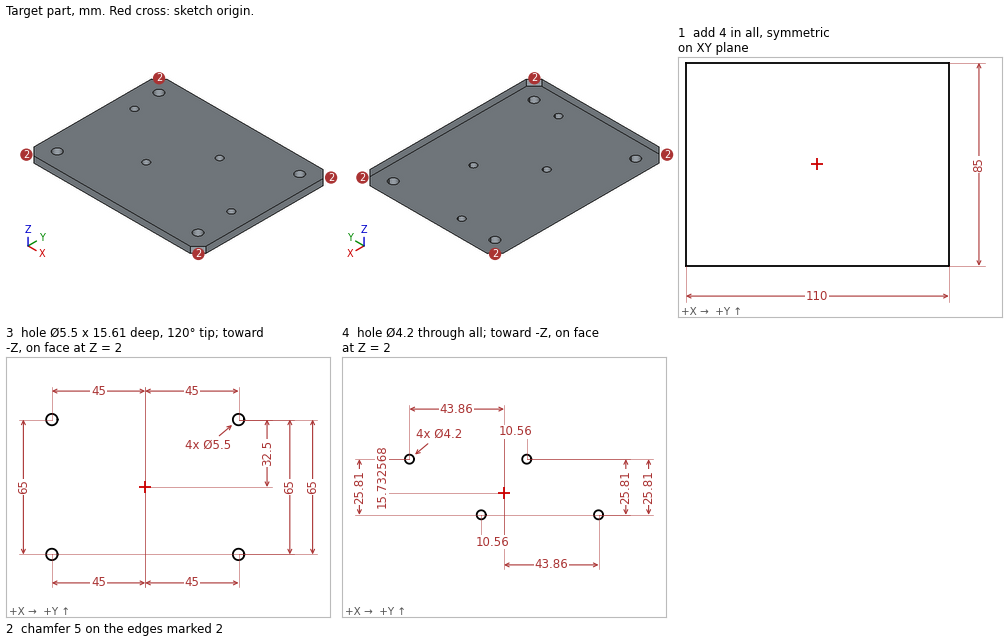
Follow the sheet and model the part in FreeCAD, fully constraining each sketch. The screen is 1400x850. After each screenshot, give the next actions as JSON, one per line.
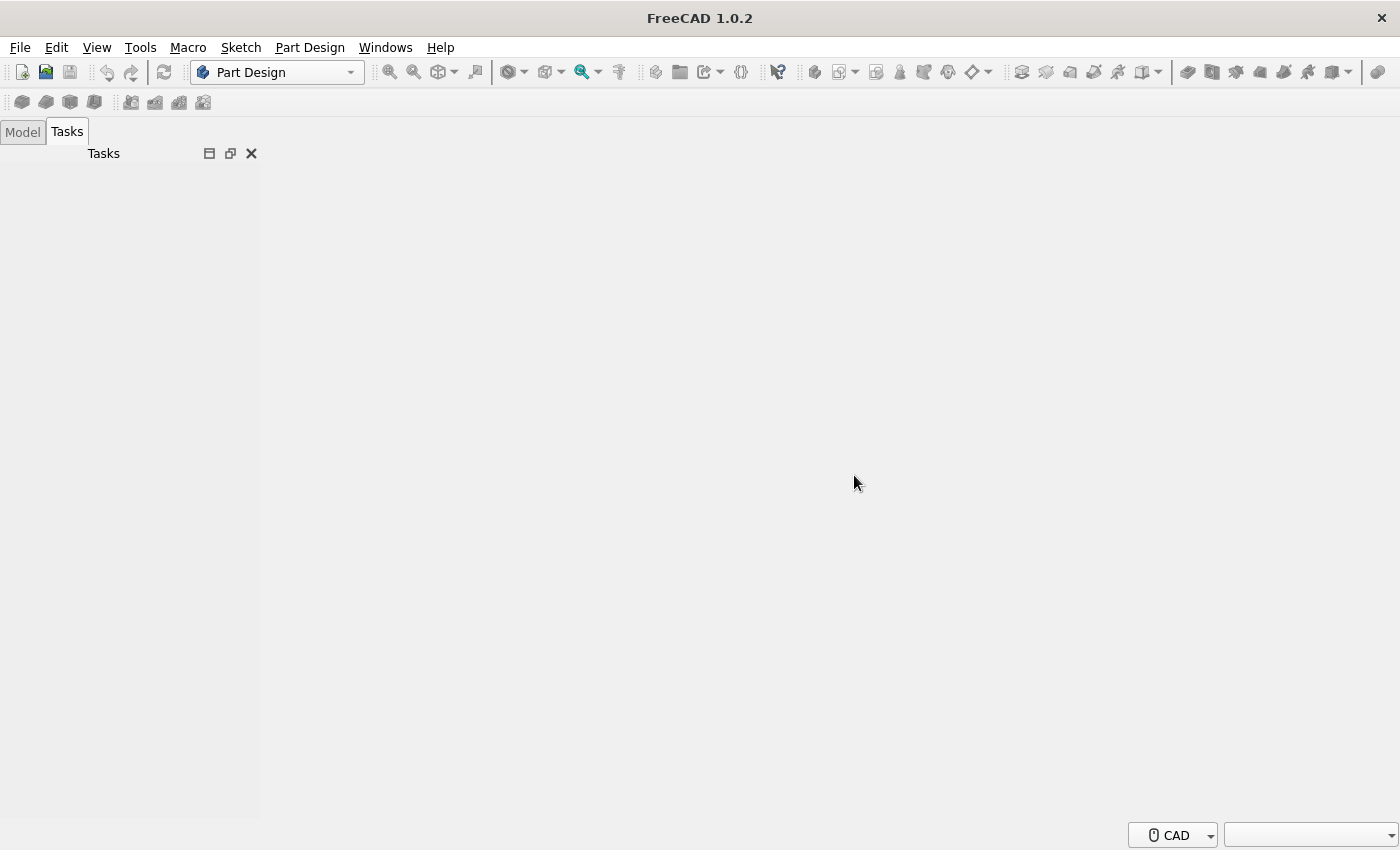
{"action": "left_click", "coordinate": [22, 72]}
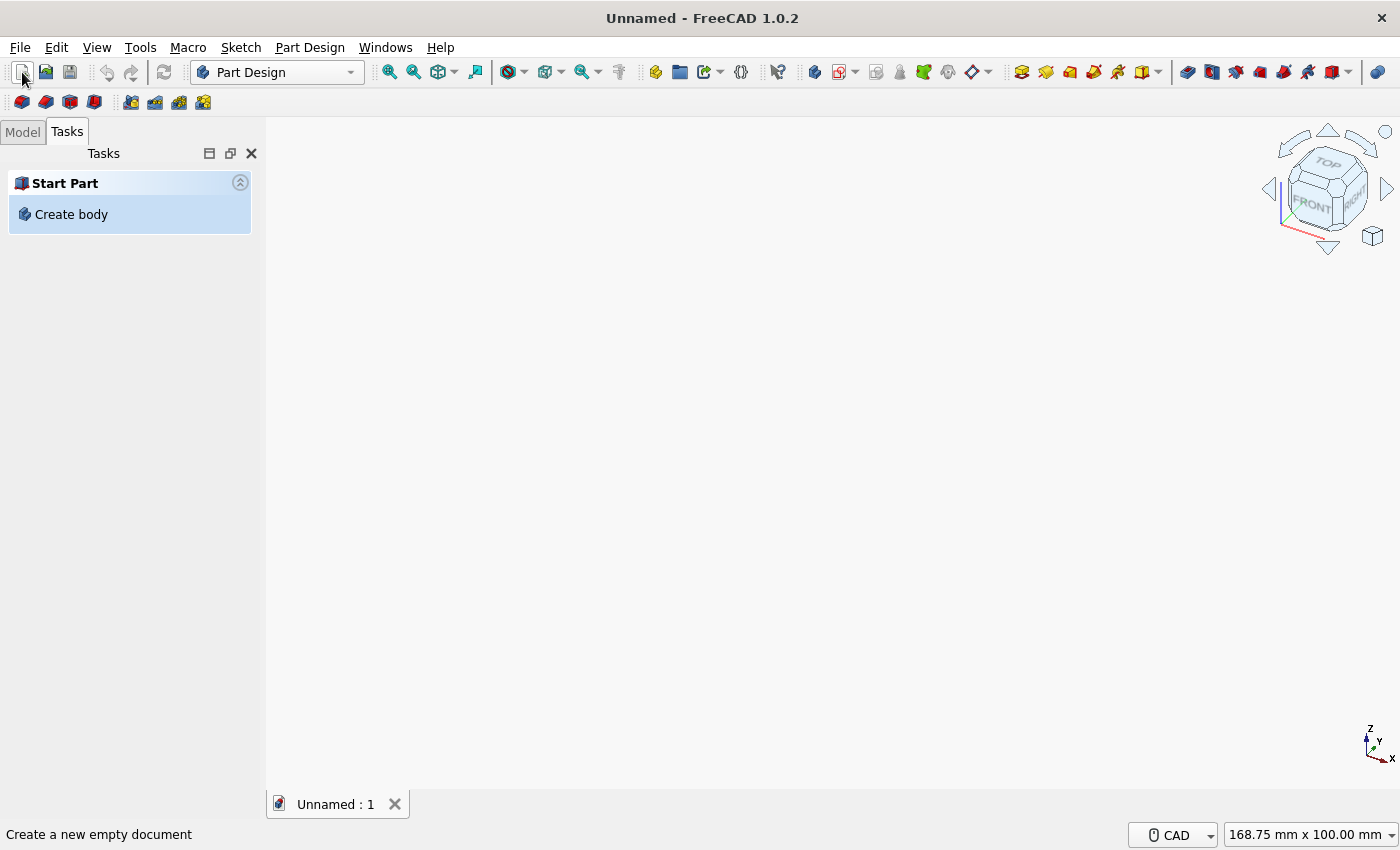
{"action": "left_click", "coordinate": [840, 72]}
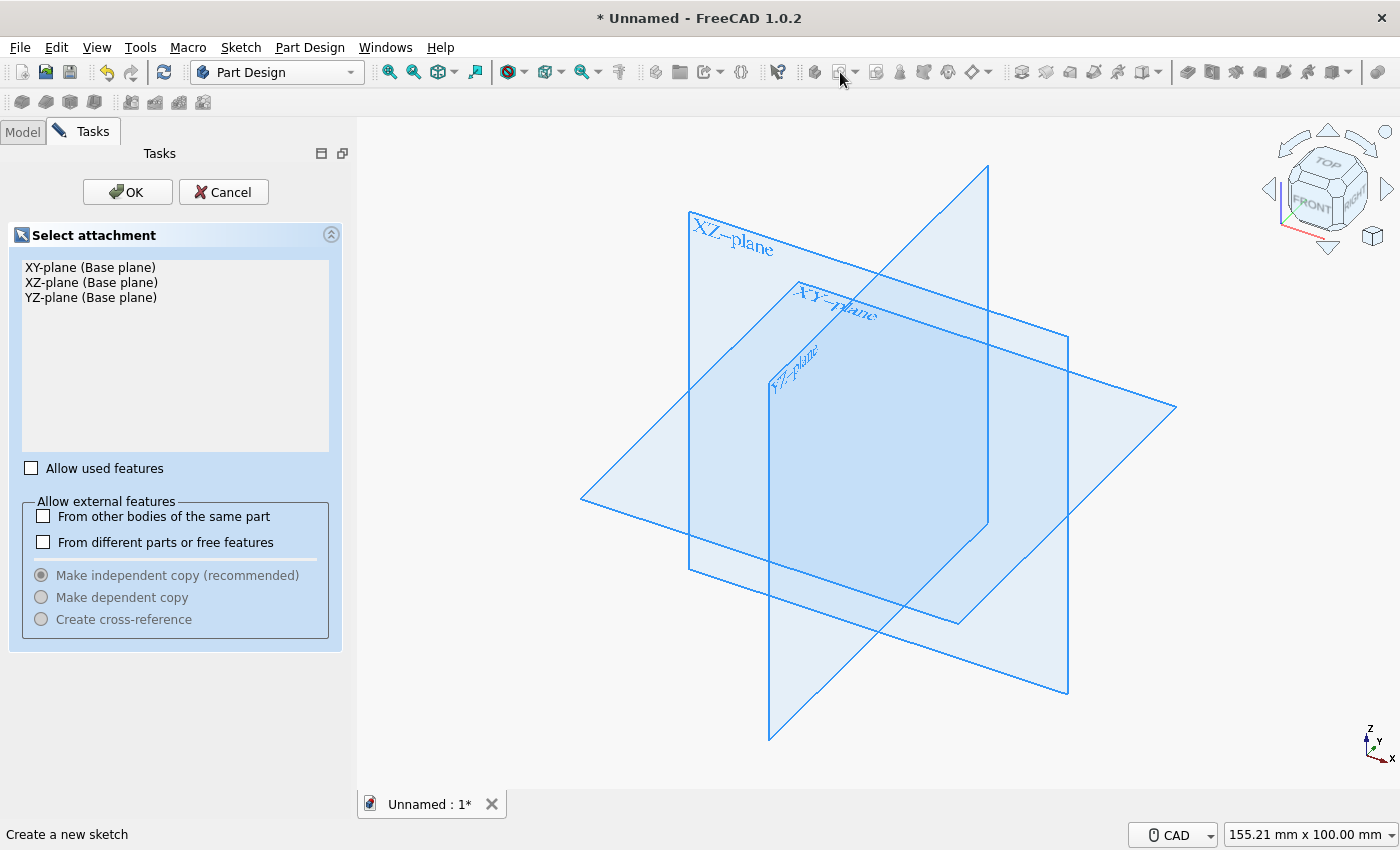
{"action": "left_click", "coordinate": [82, 268]}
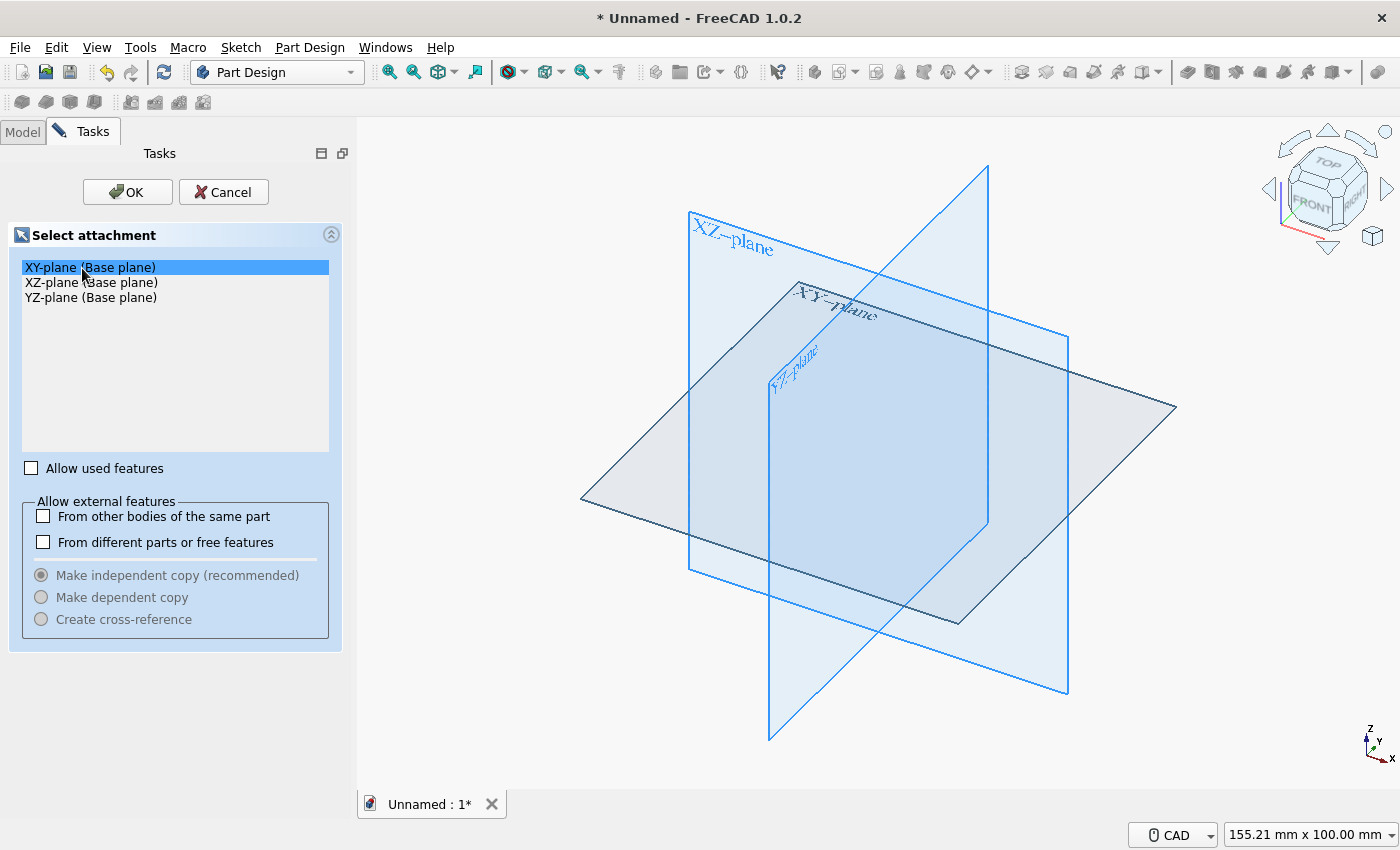
{"action": "left_click", "coordinate": [128, 192]}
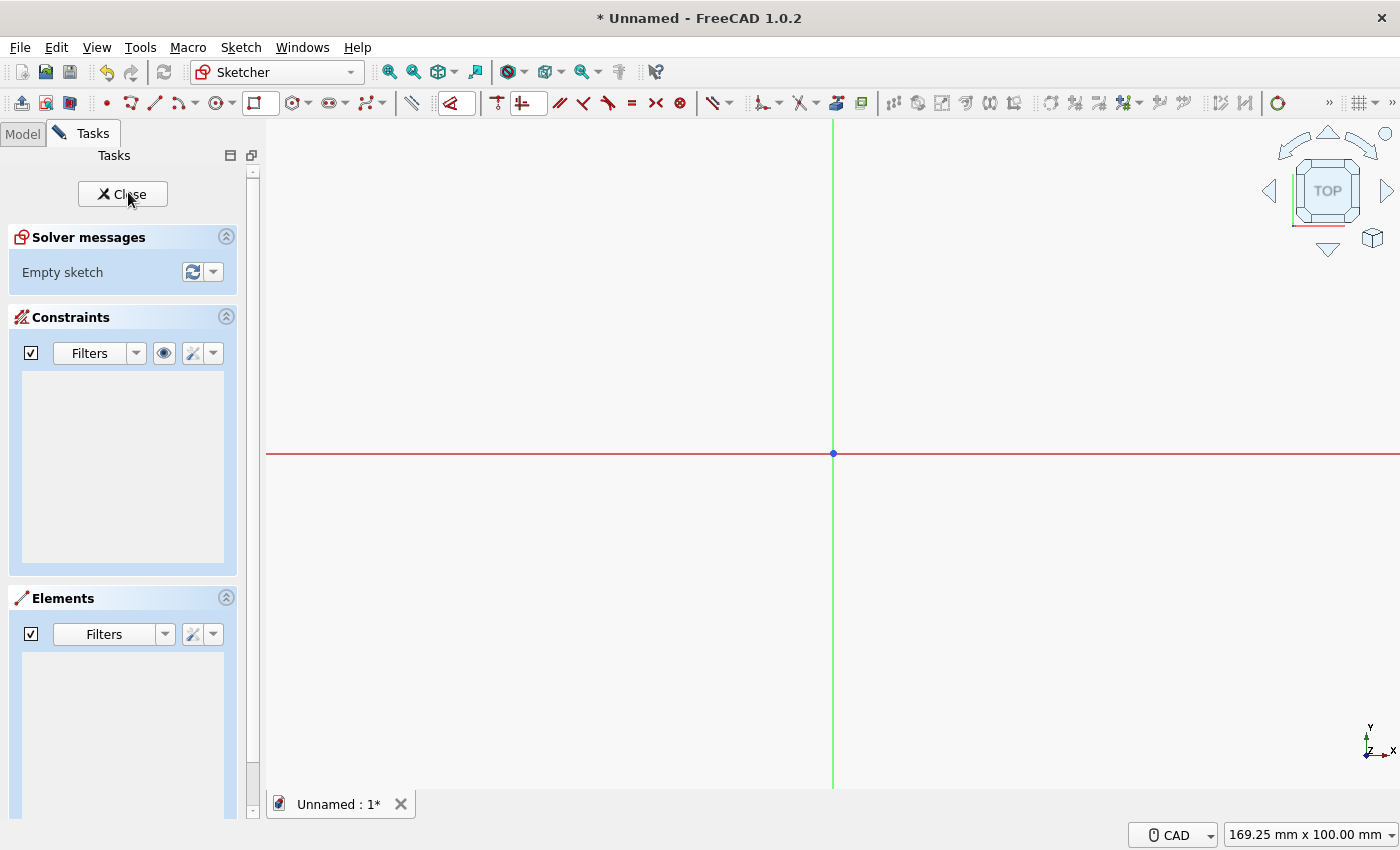
{"action": "scroll", "coordinate": [455, 454], "scroll_direction": "down", "scroll_amount": 1}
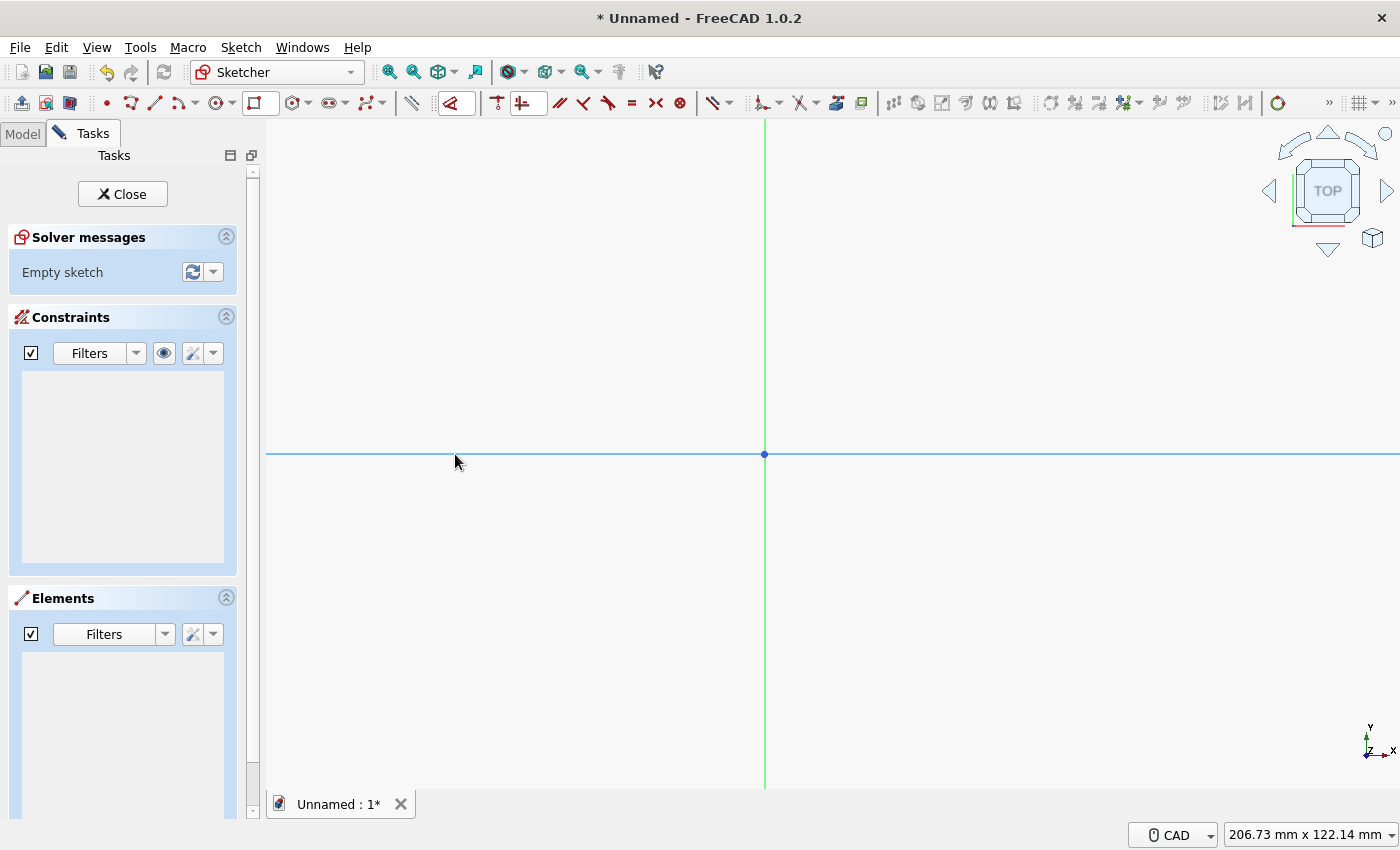
{"action": "key", "text": "g v"}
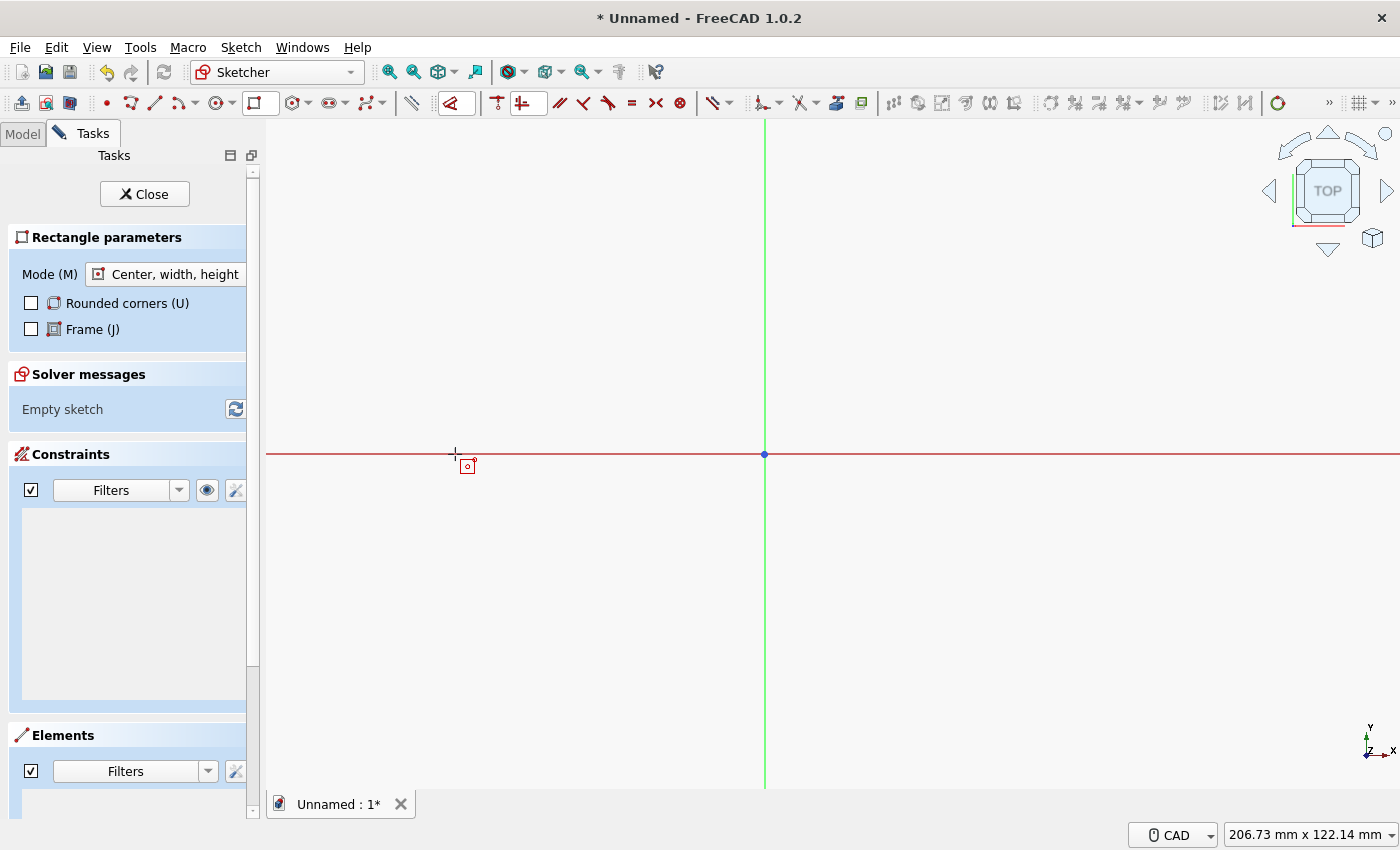
{"action": "left_click", "coordinate": [765, 454]}
{"action": "mouse_move", "coordinate": [1066, 221]}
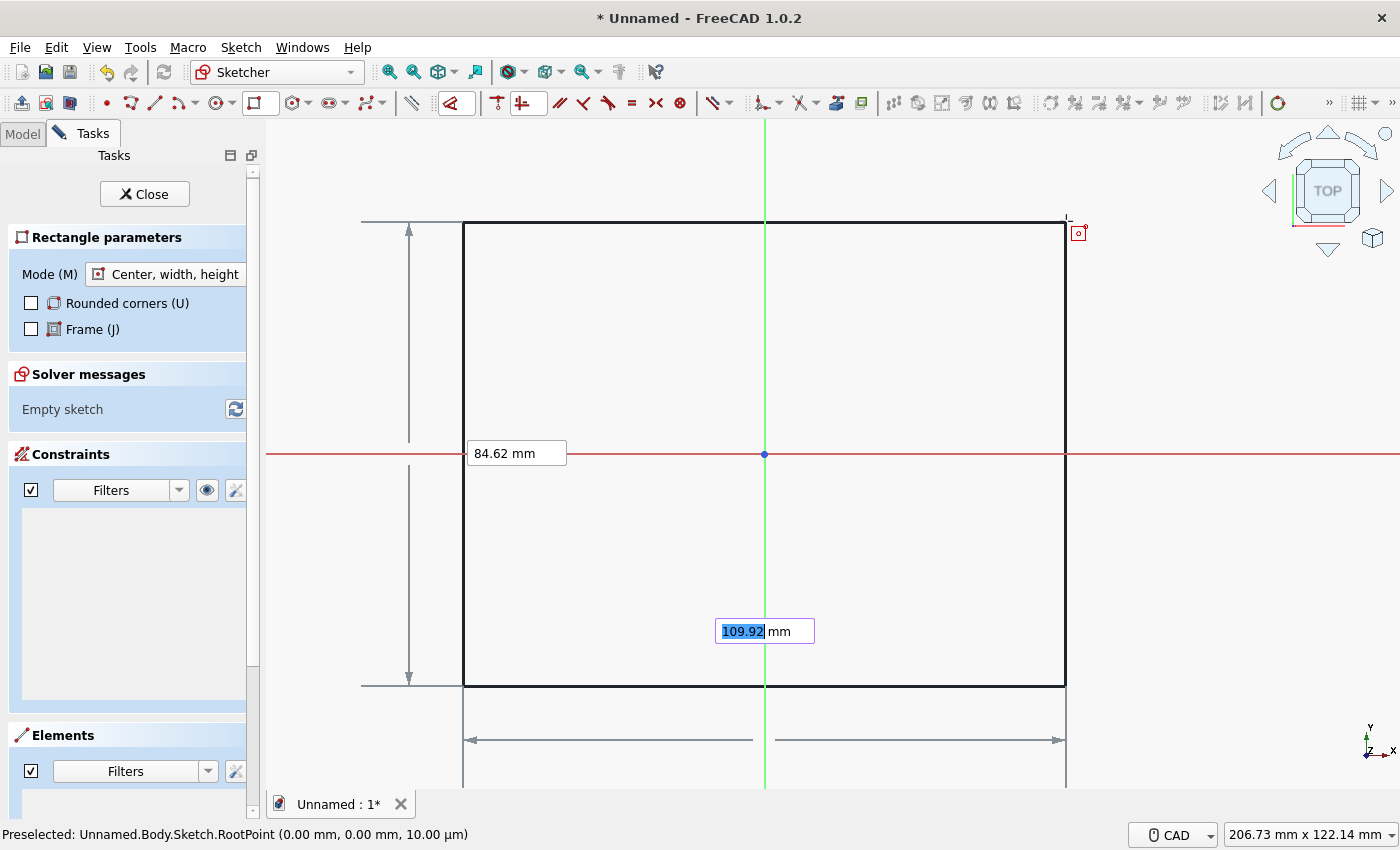
{"action": "type", "text": "110"}
{"action": "key", "text": "Tab"}
{"action": "type", "text": "85"}
{"action": "key", "text": "Return"}
{"action": "key", "text": "Escape"}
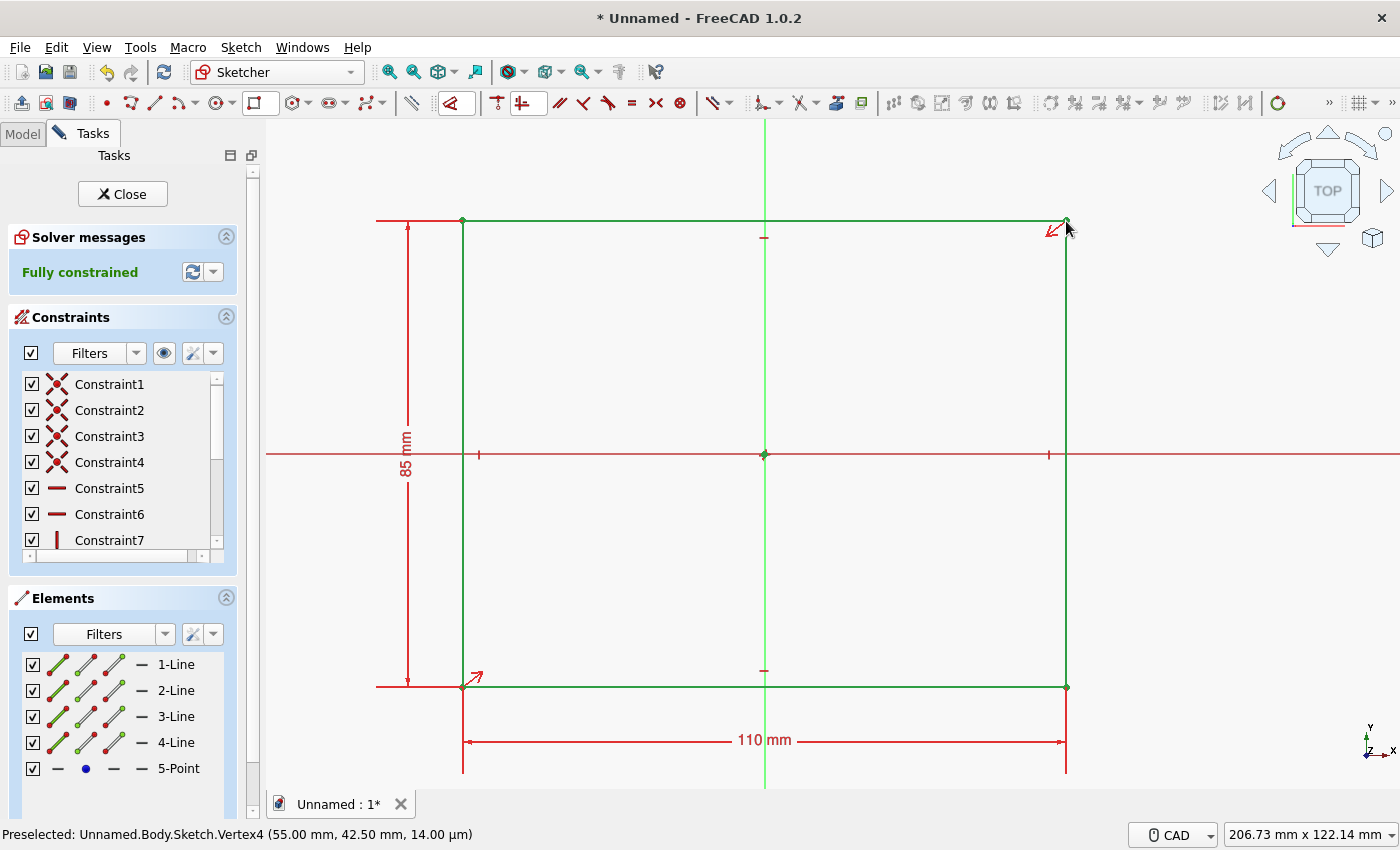
{"action": "left_click", "coordinate": [123, 194]}